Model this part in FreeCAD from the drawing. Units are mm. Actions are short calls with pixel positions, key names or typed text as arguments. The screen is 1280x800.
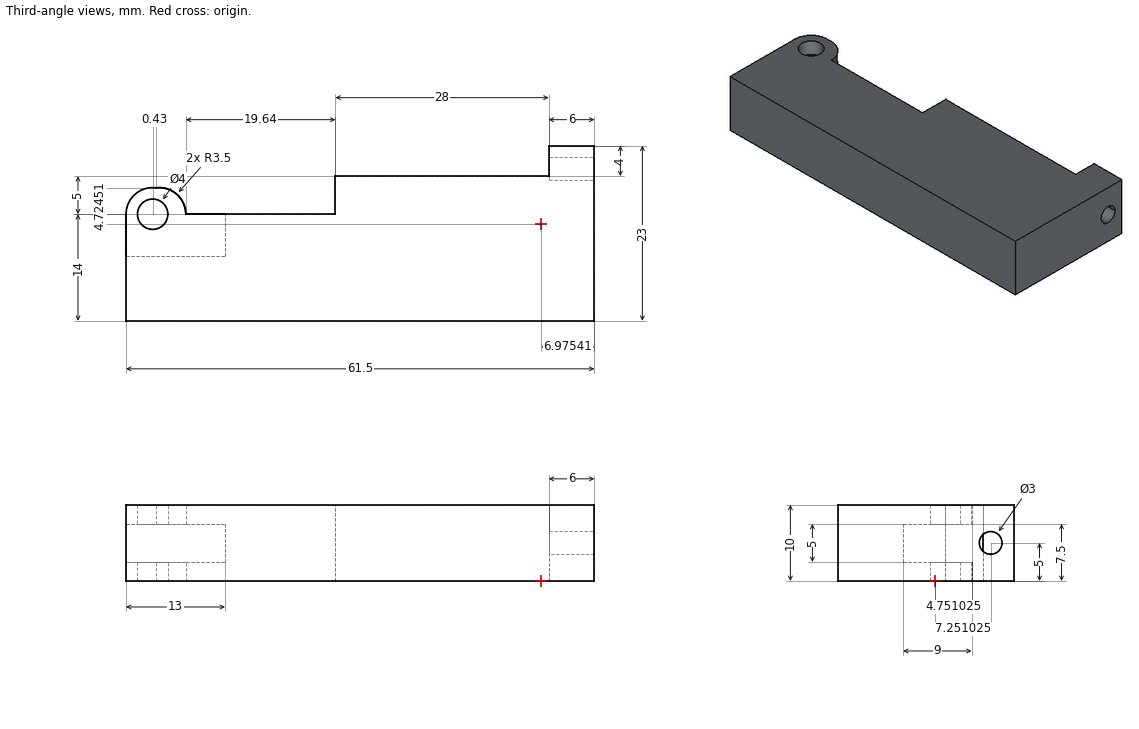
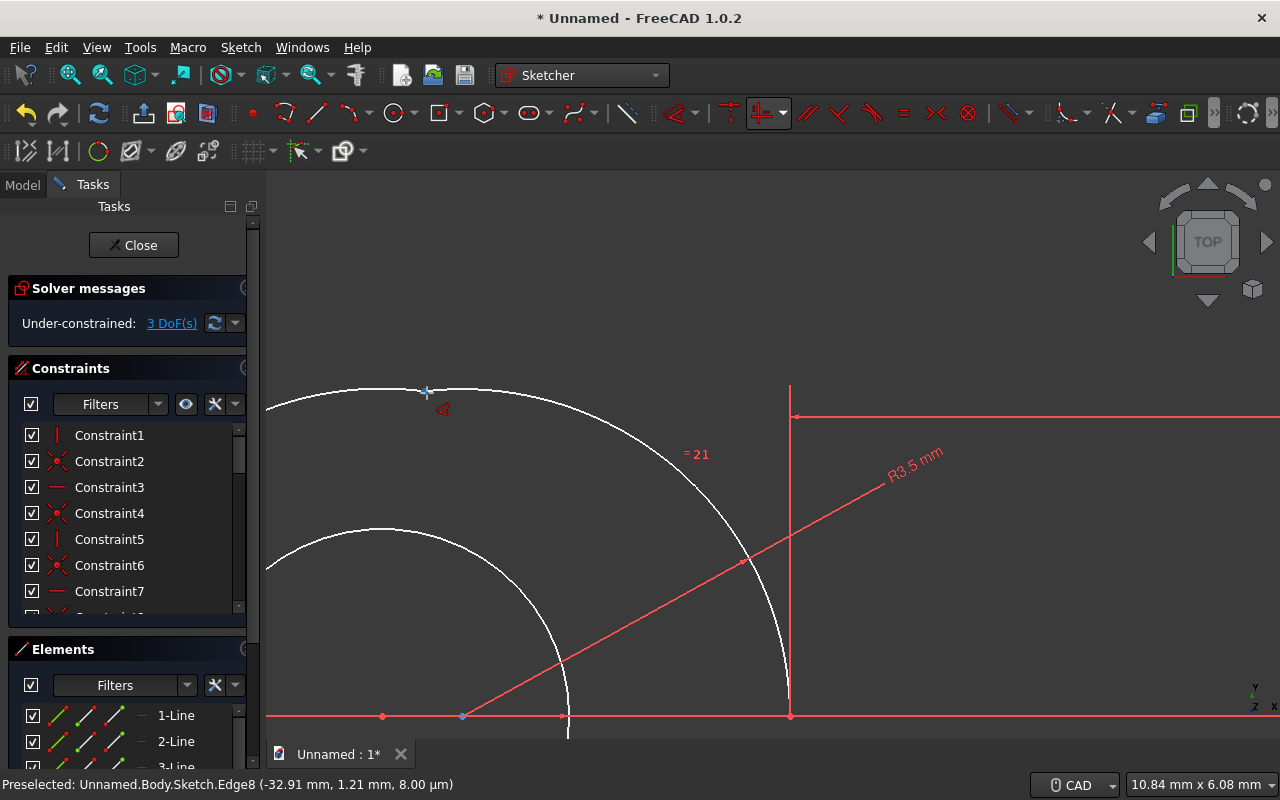
click(424, 391)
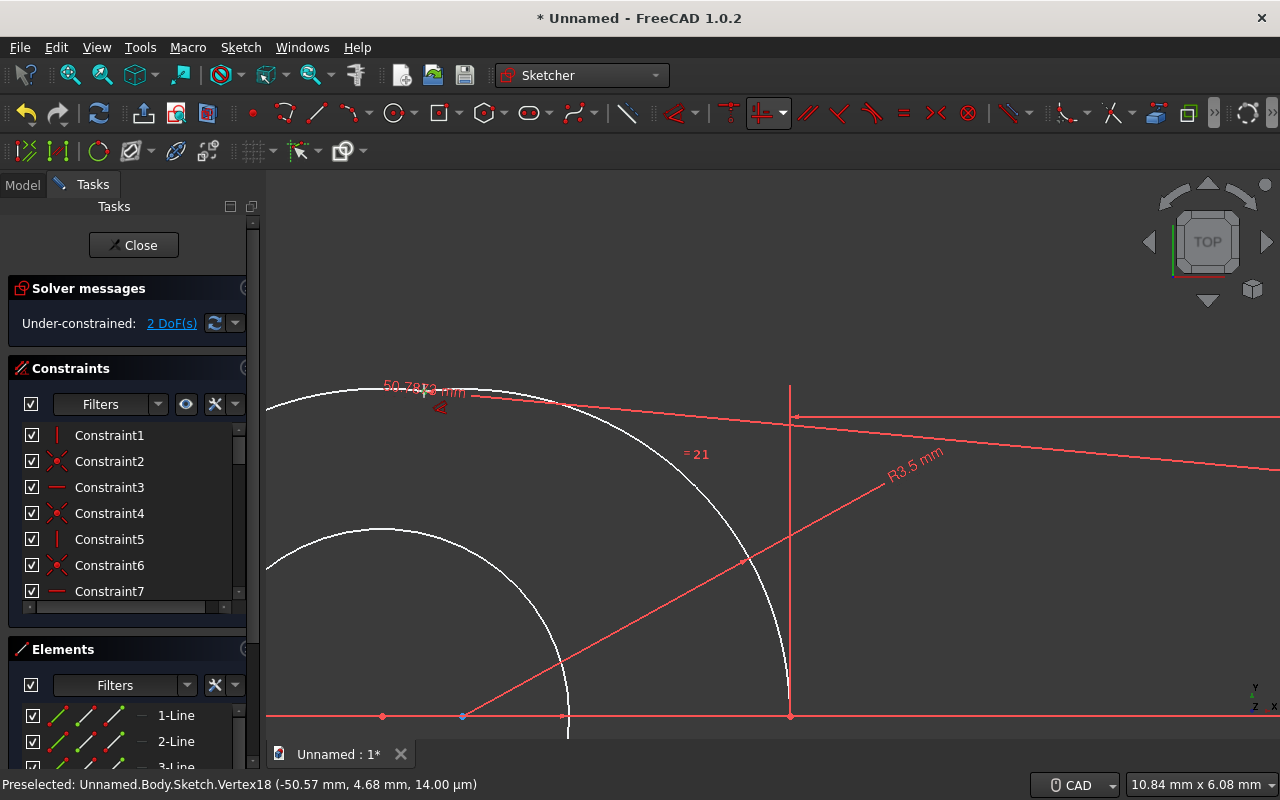
scroll(427, 393, down, 11)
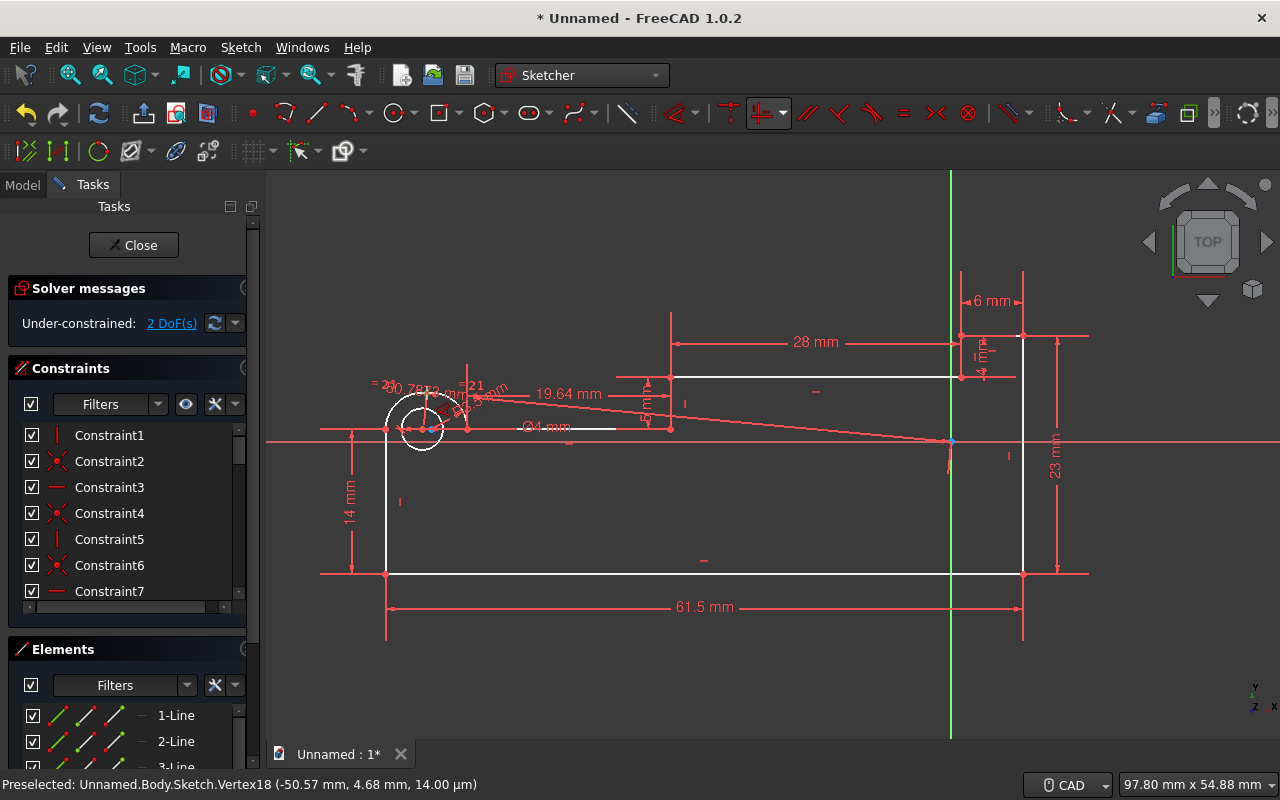
scroll(422, 429, up, 11)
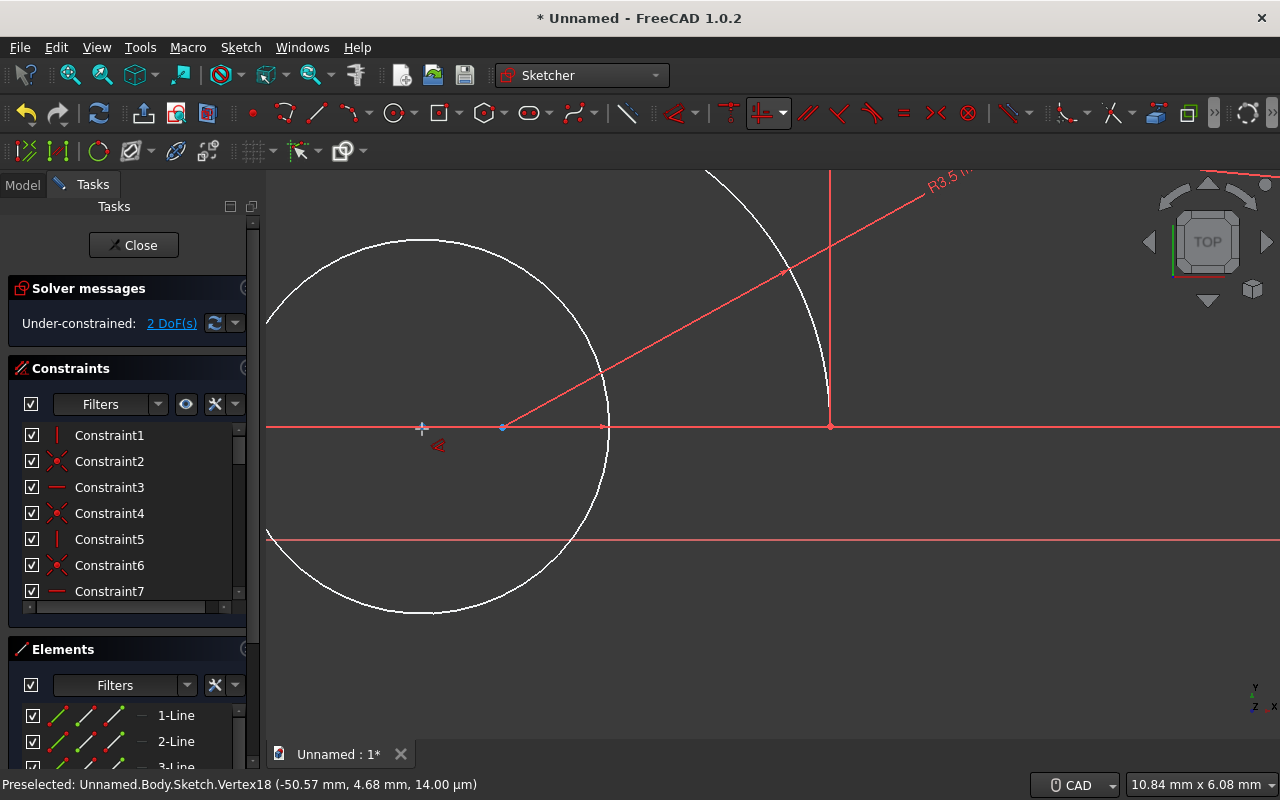
click(422, 427)
click(443, 461)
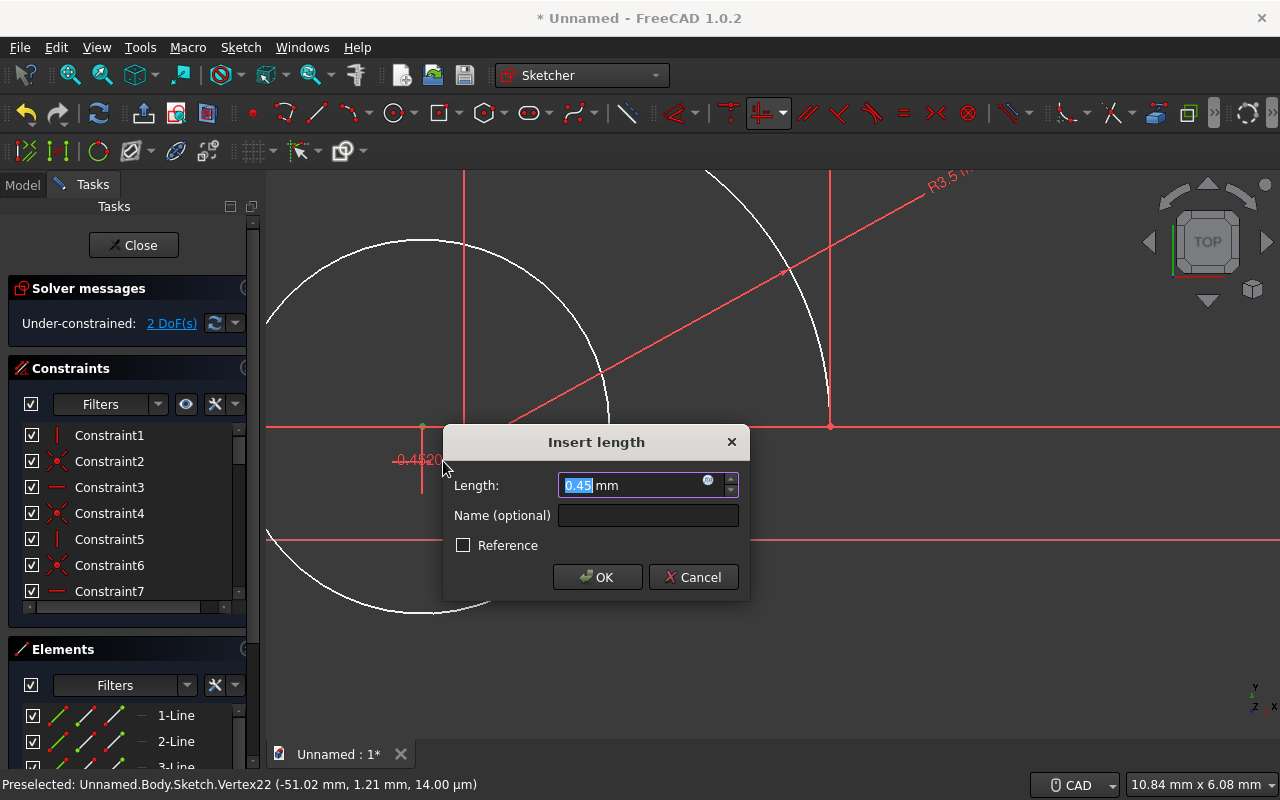
text(0.43)
key(Return)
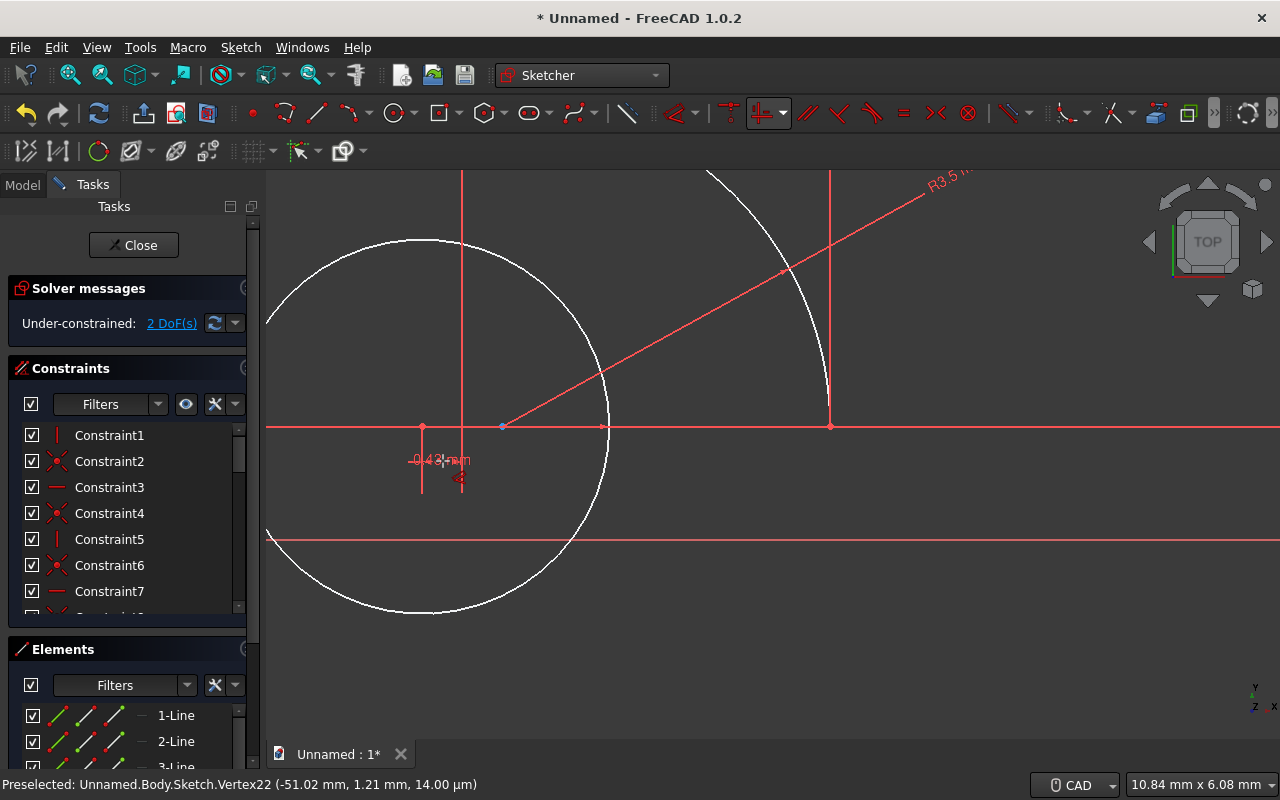
scroll(422, 429, down, 11)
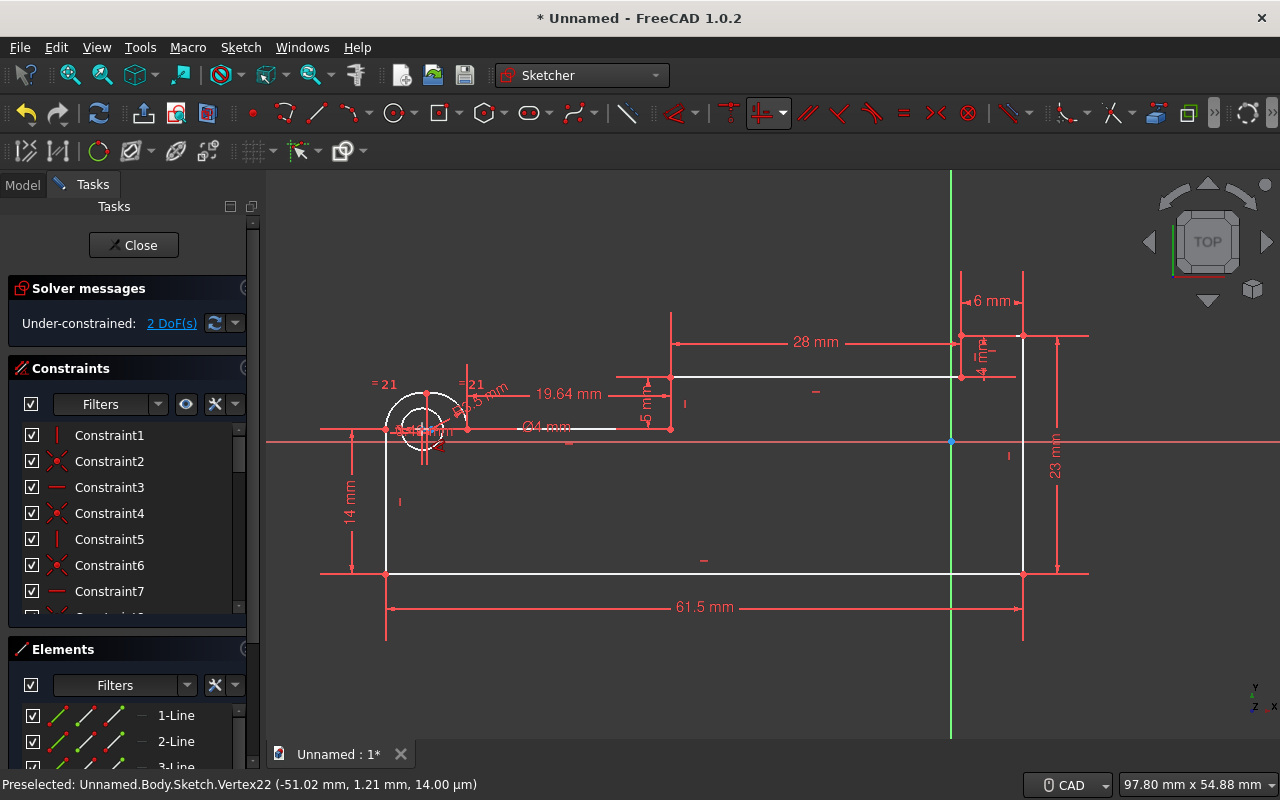
click(1023, 574)
click(987, 608)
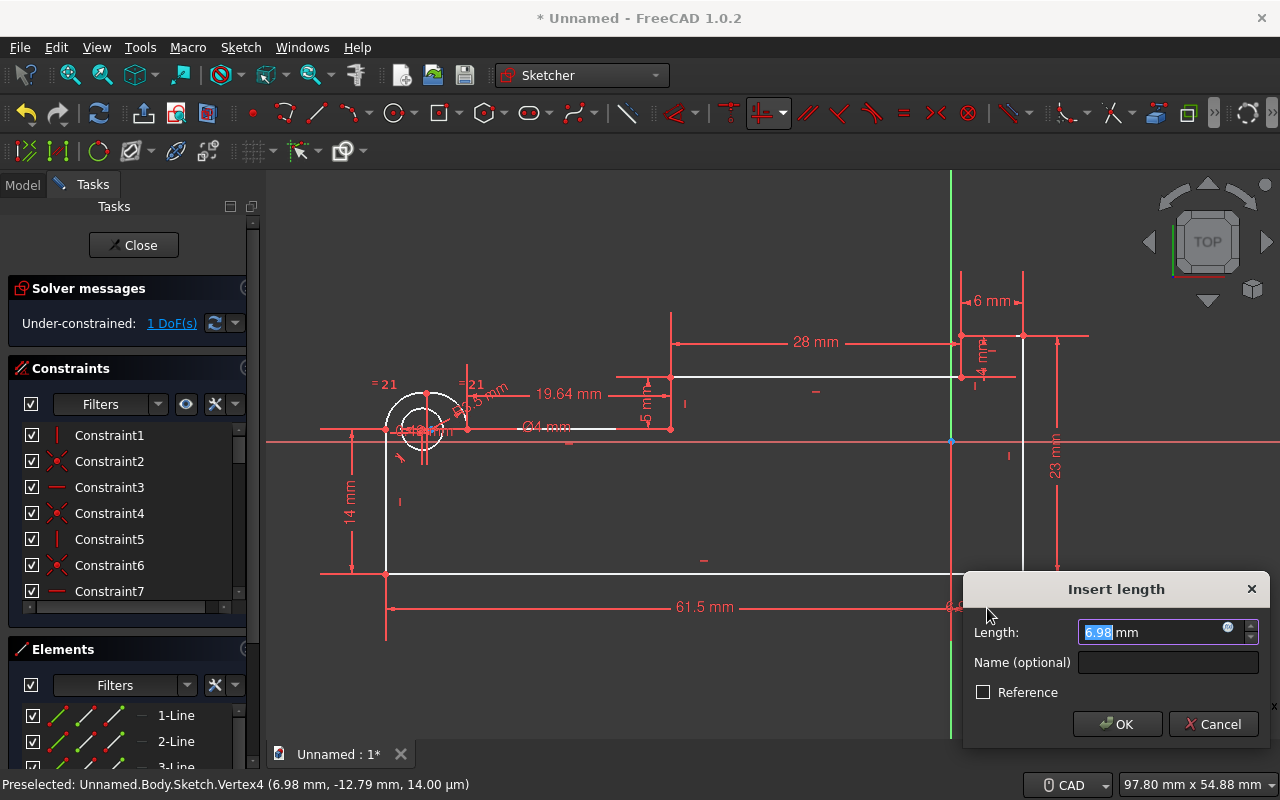
text(6.97541)
key(Return)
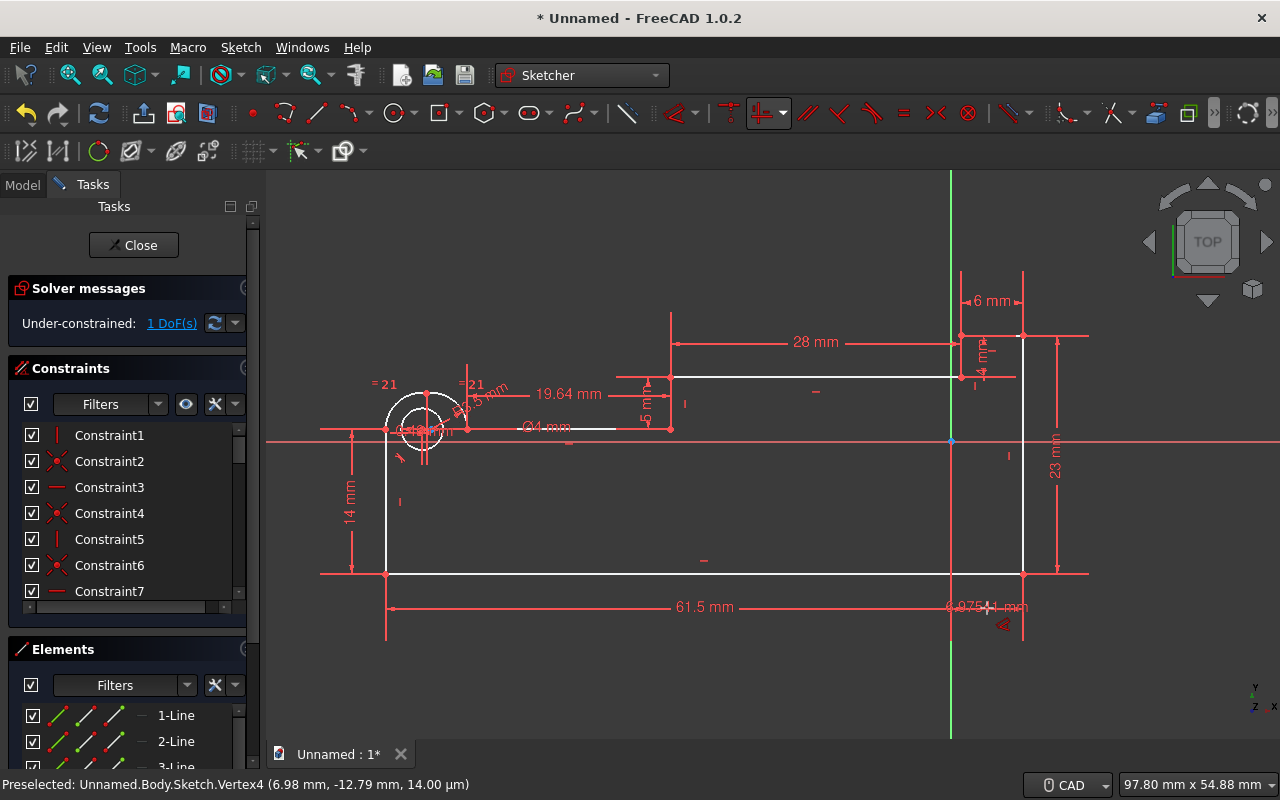
click(427, 393)
click(985, 417)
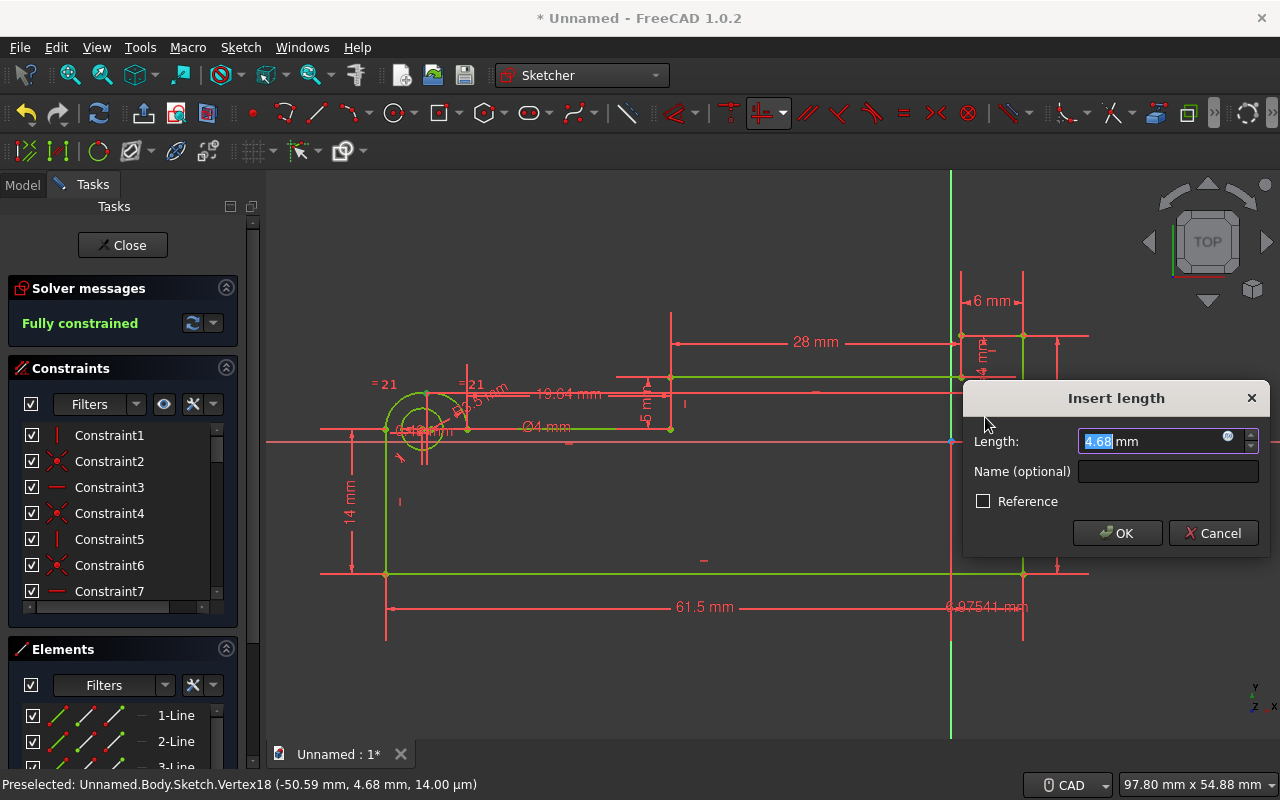
text(4.72451)
key(Return)
key(Escape)